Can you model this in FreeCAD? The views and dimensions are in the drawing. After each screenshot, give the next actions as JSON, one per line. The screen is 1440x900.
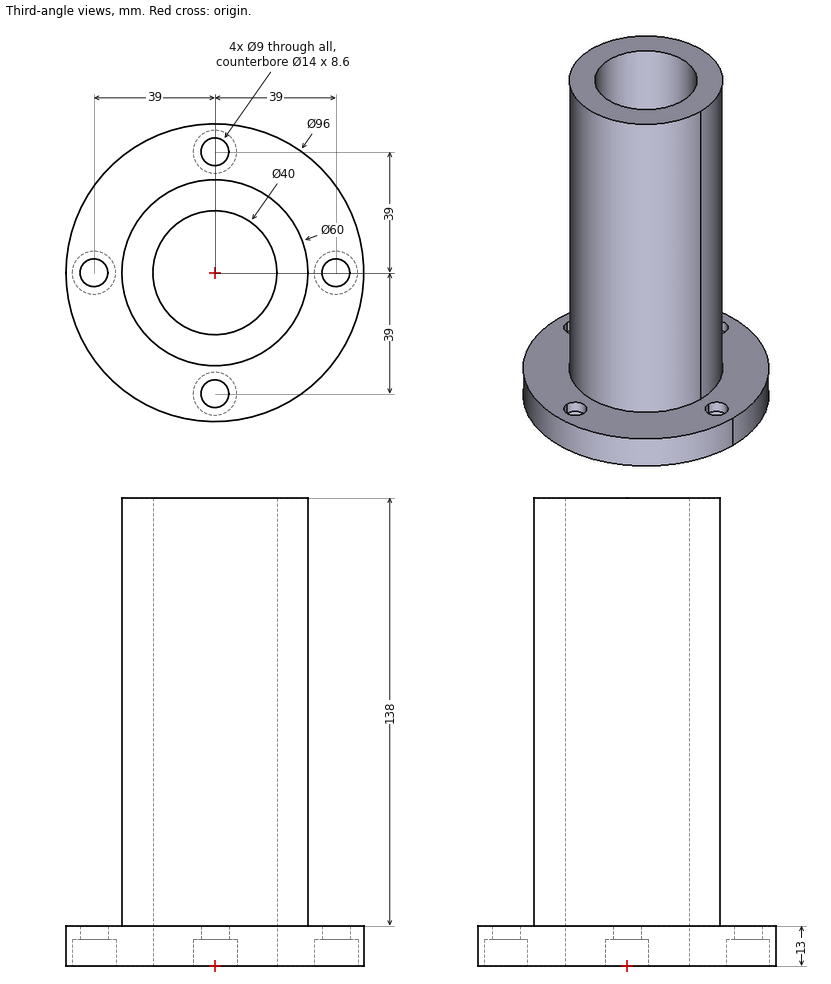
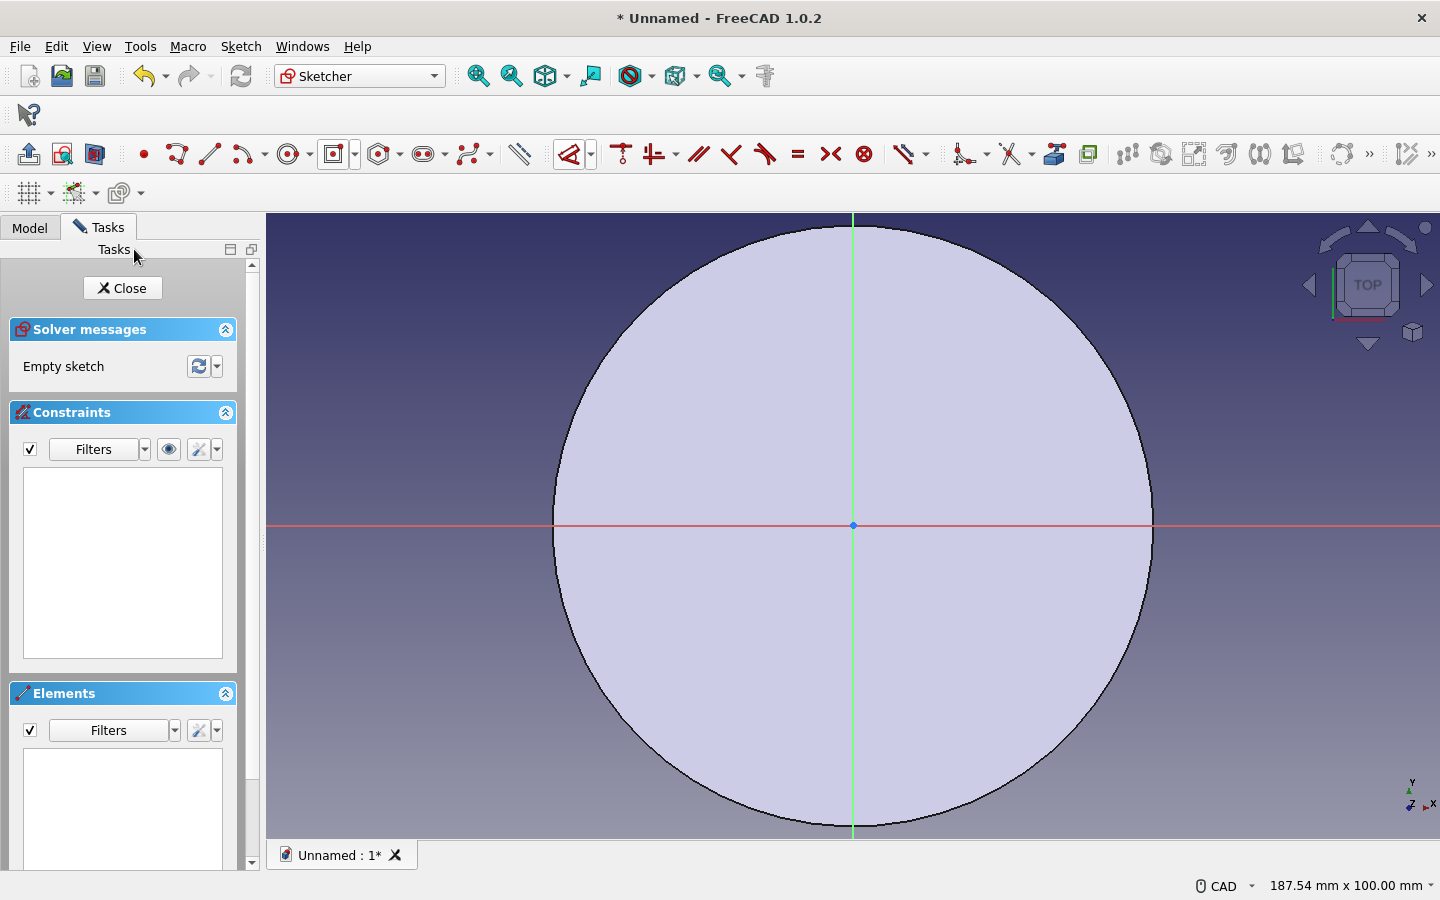
{"action": "scroll", "coordinate": [645, 526], "scroll_direction": "down", "scroll_amount": 2}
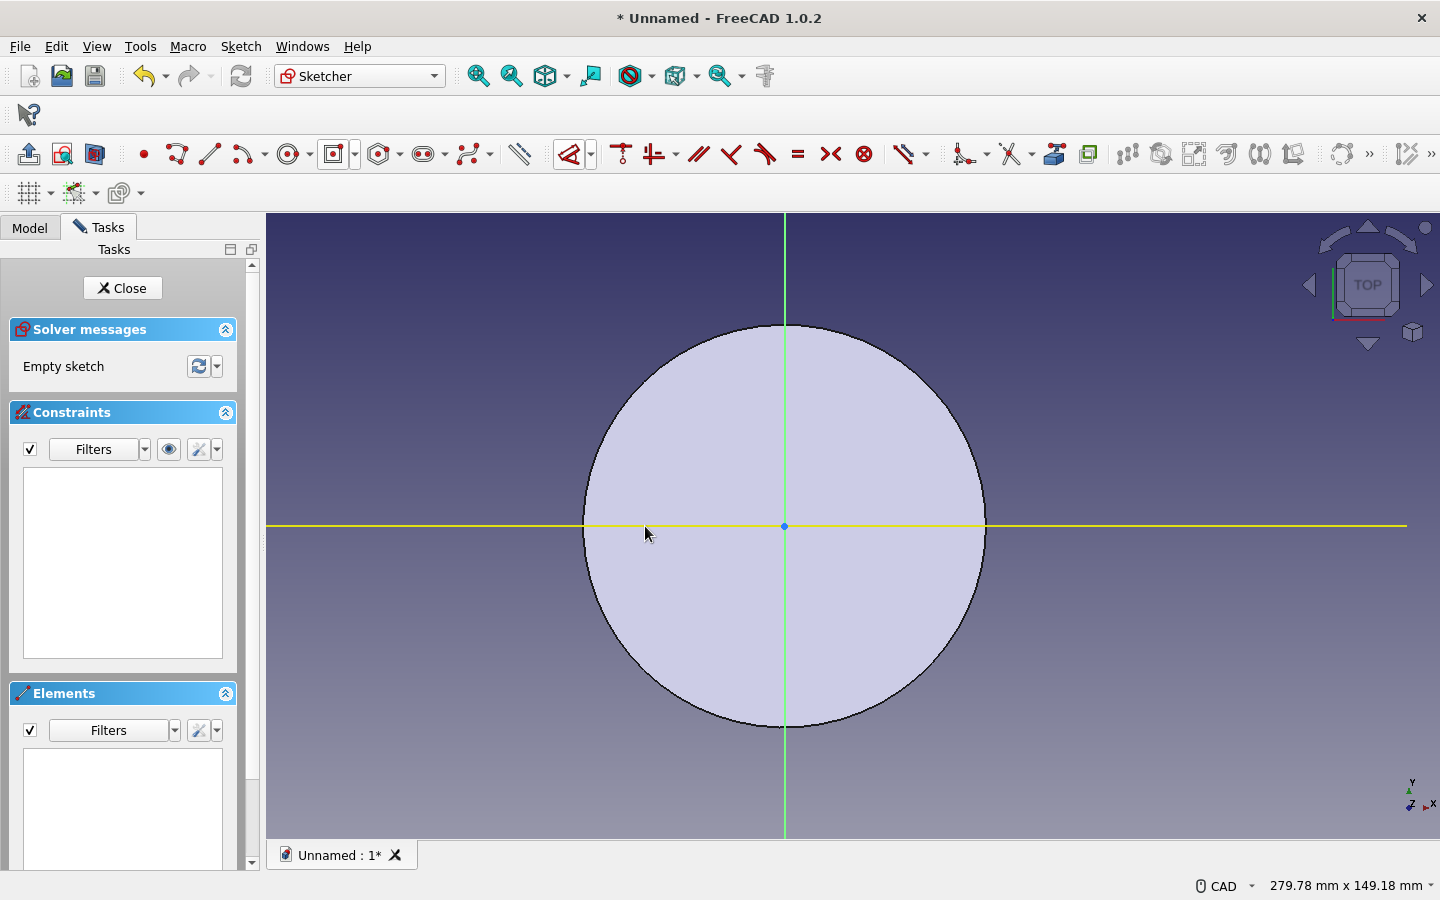
{"action": "left_click", "coordinate": [288, 154]}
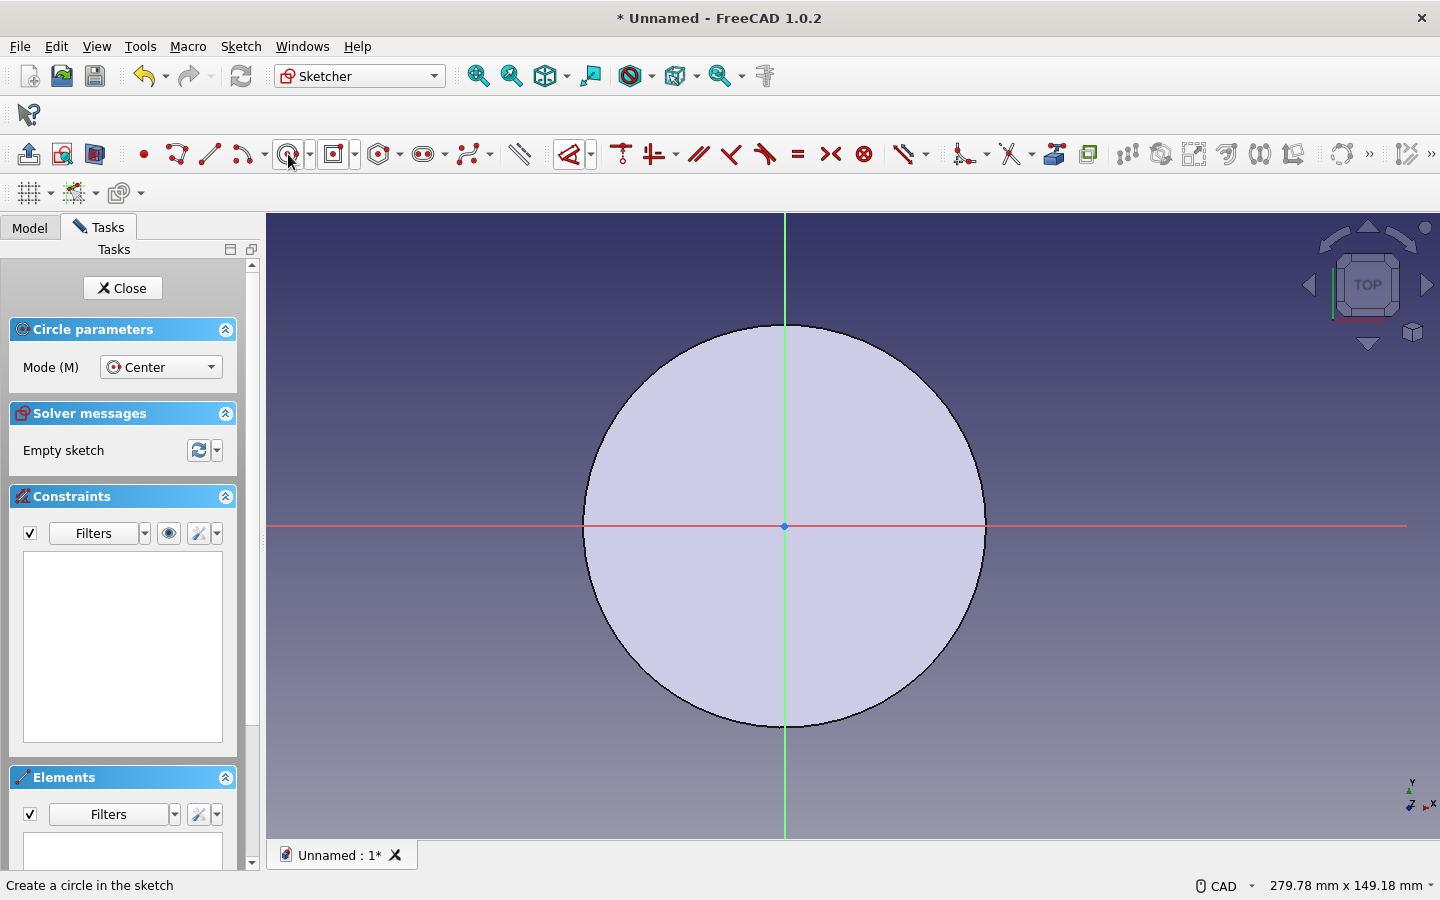
{"action": "left_click", "coordinate": [785, 363]}
{"action": "mouse_move", "coordinate": [802, 356]}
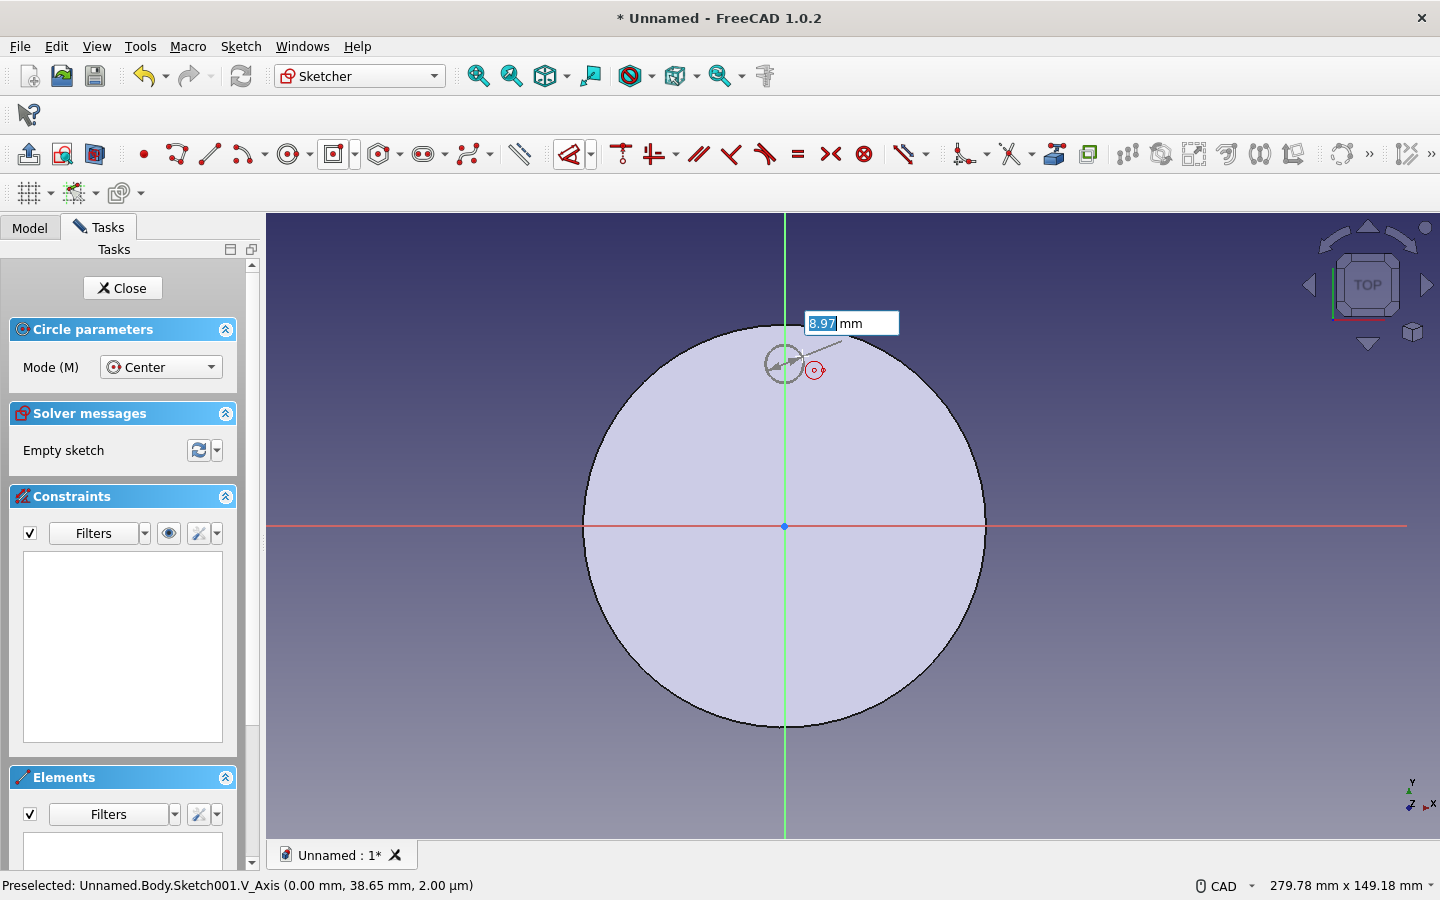
{"action": "type", "text": "9"}
{"action": "key", "text": "Return"}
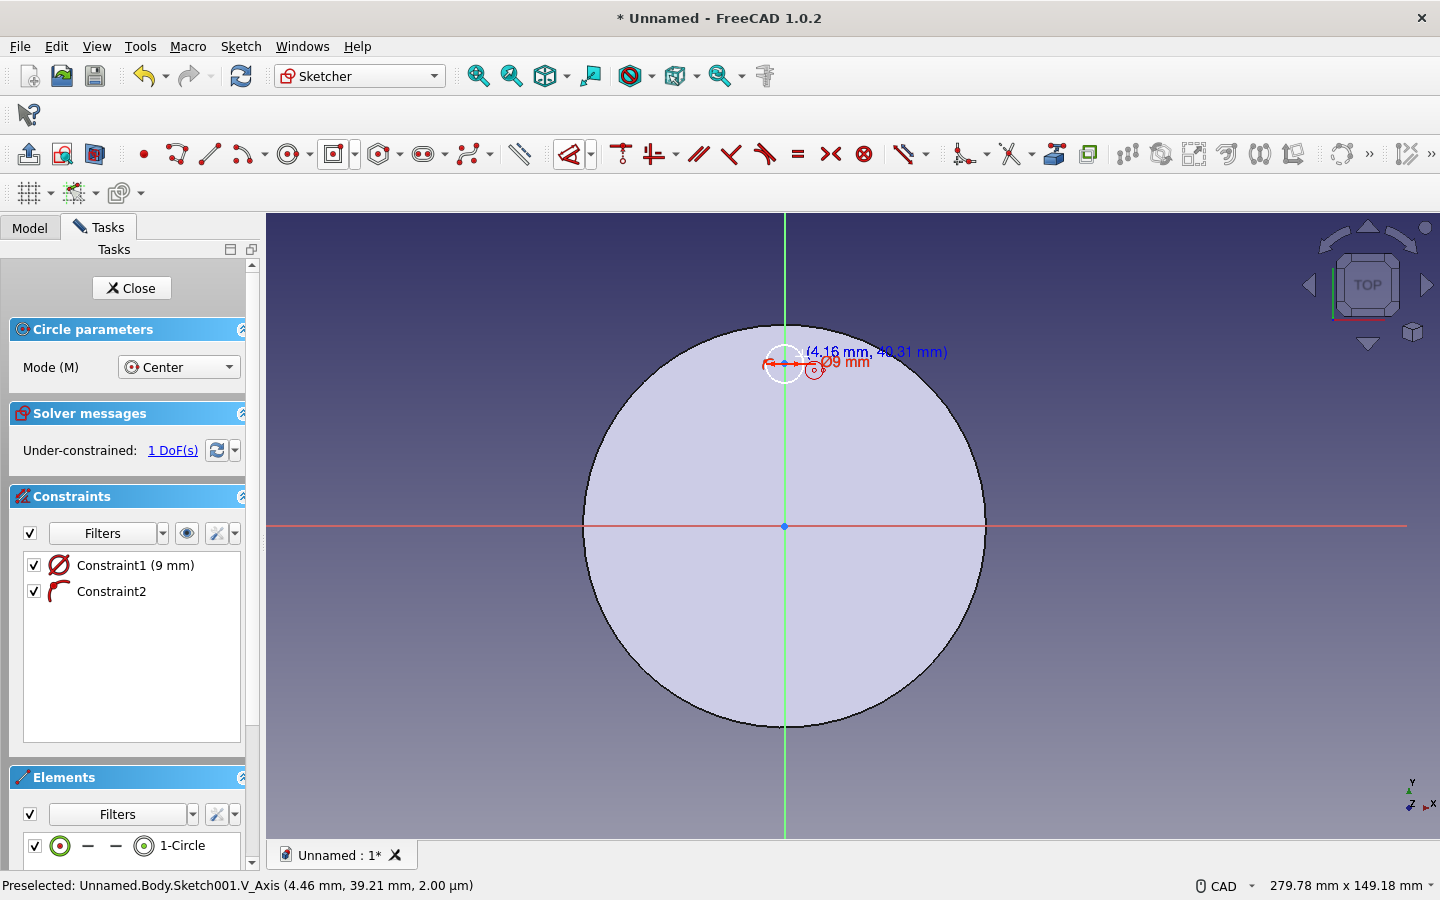
{"action": "left_click", "coordinate": [948, 526]}
{"action": "mouse_move", "coordinate": [955, 508]}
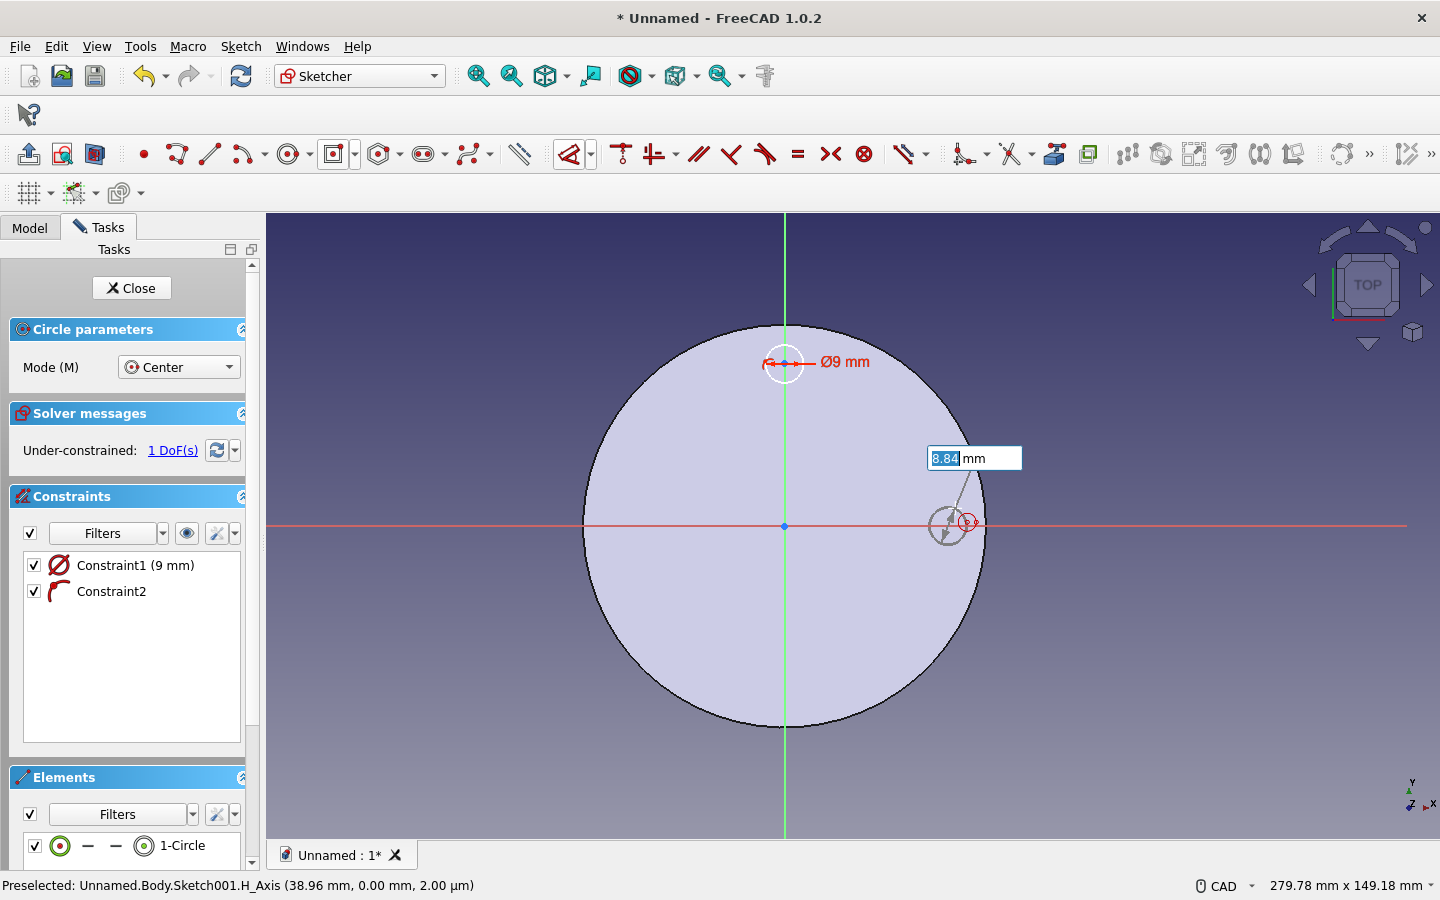
{"action": "type", "text": "9"}
{"action": "key", "text": "Return"}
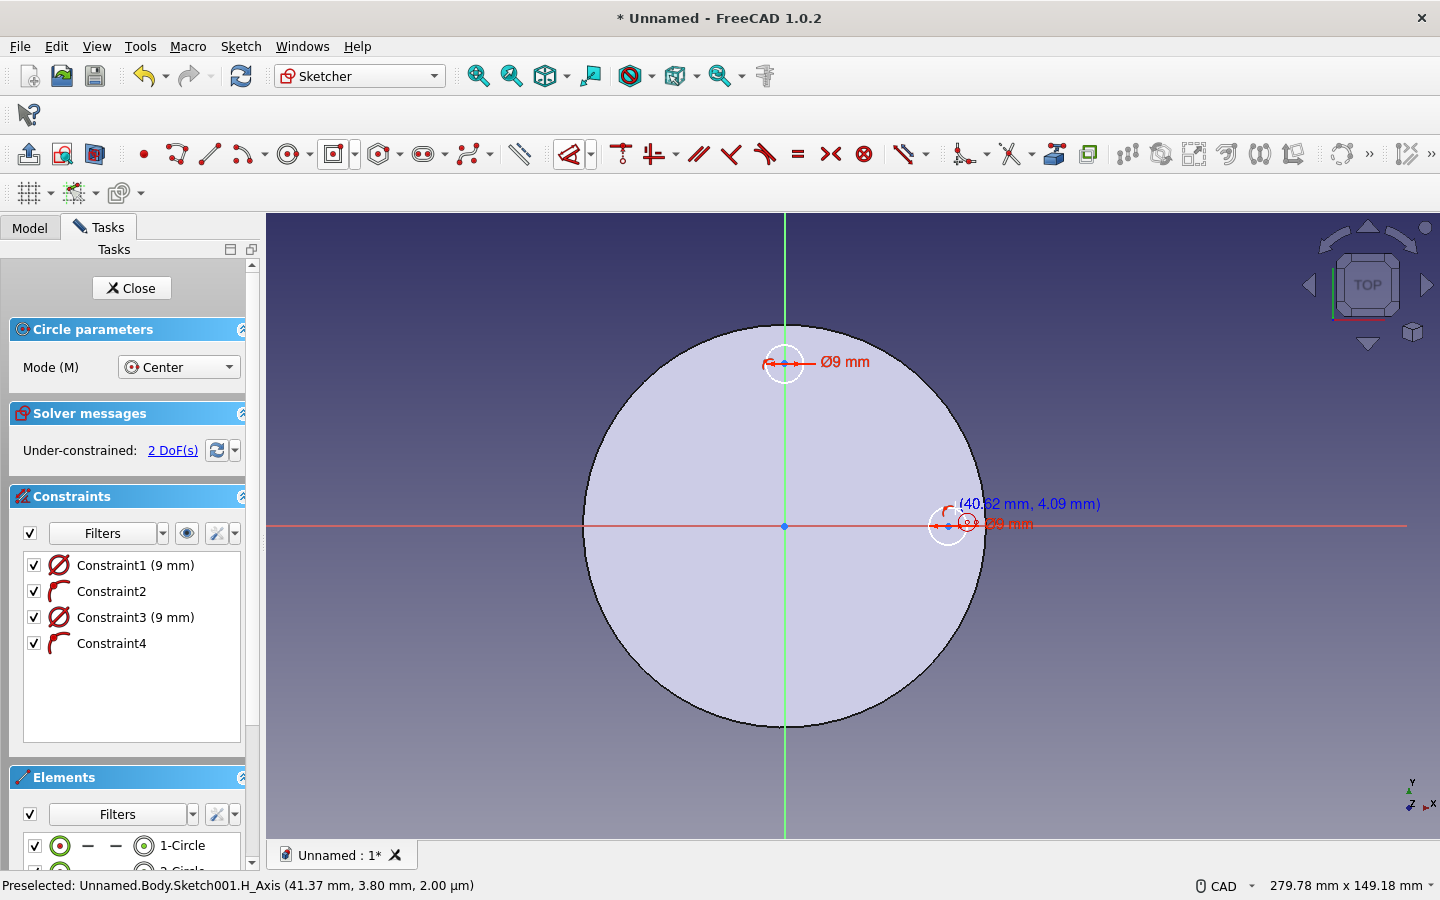
{"action": "left_click", "coordinate": [785, 690]}
{"action": "mouse_move", "coordinate": [802, 683]}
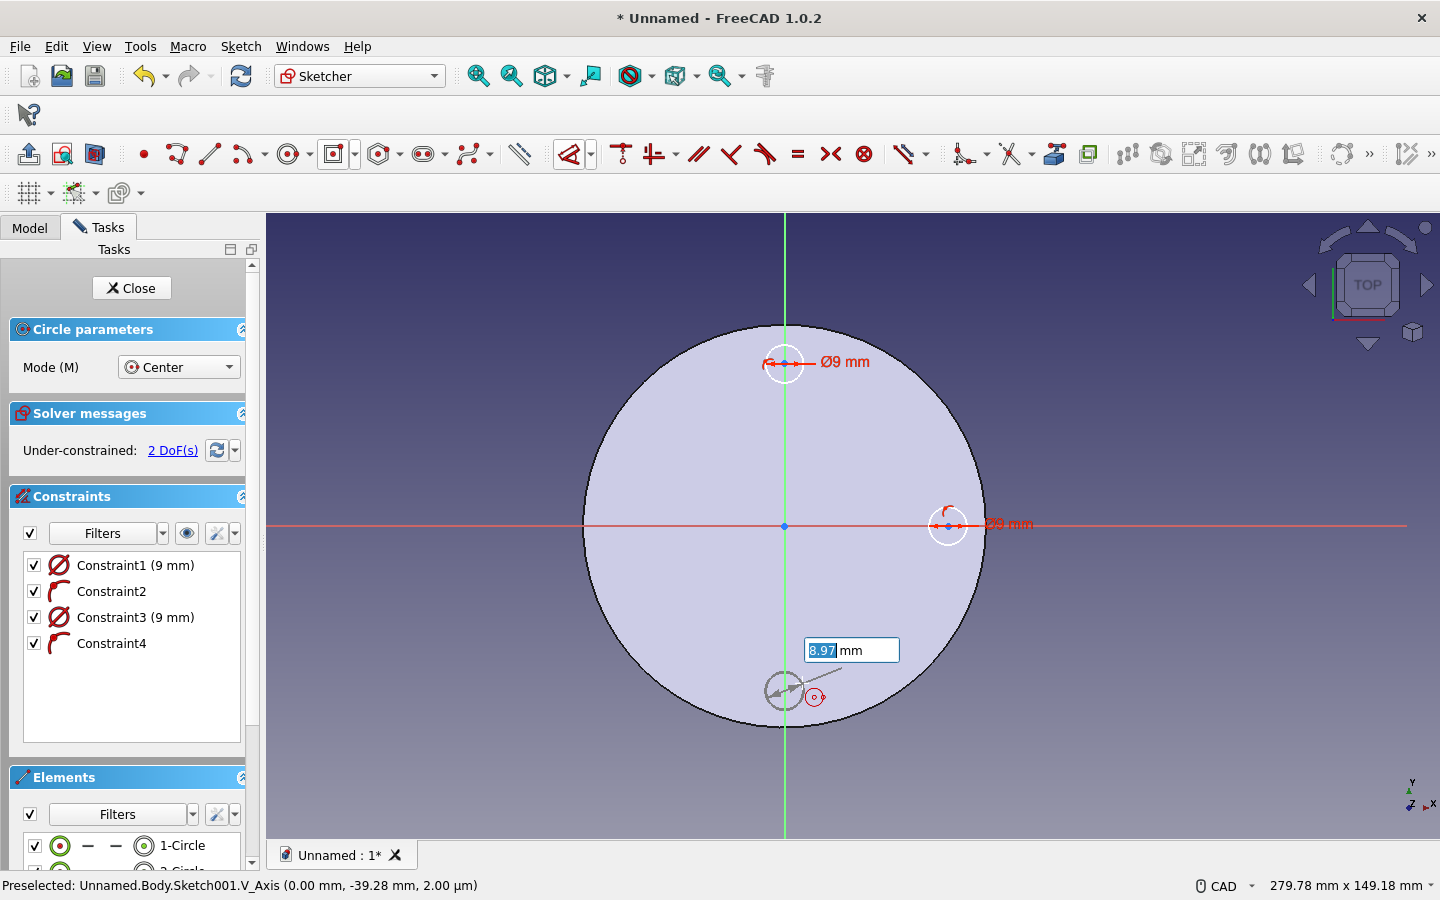
{"action": "type", "text": "9"}
{"action": "key", "text": "Return"}